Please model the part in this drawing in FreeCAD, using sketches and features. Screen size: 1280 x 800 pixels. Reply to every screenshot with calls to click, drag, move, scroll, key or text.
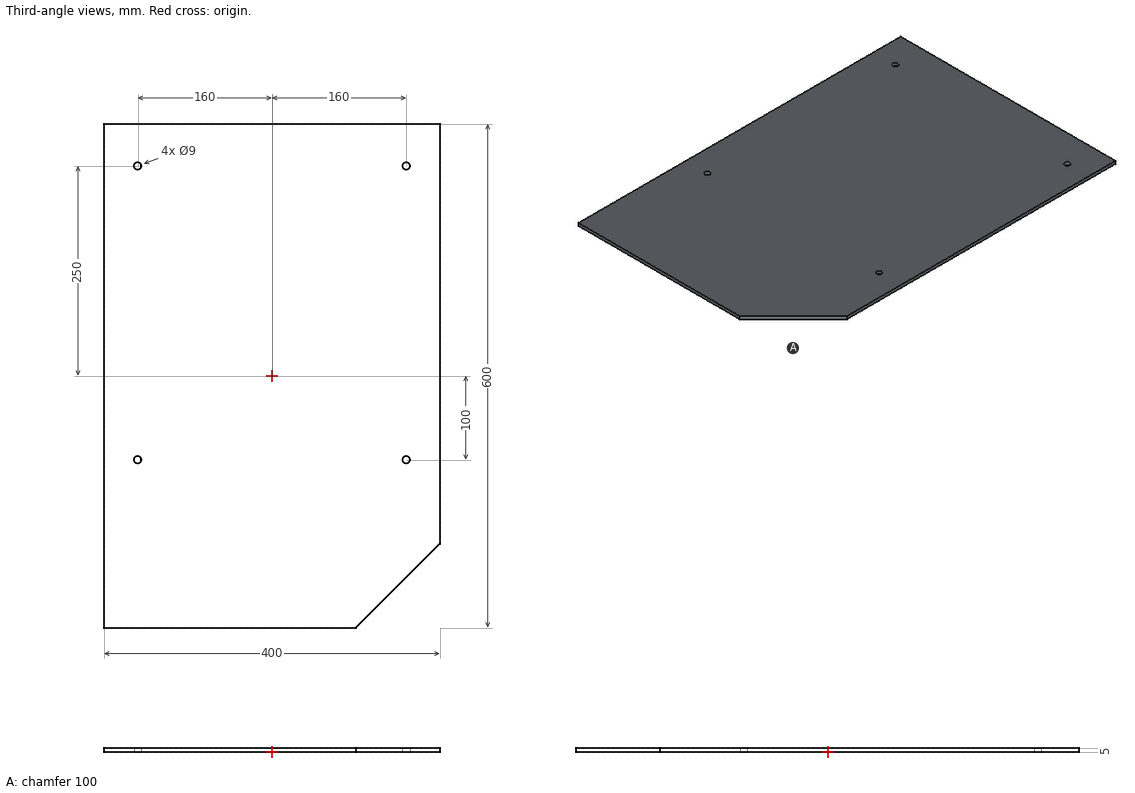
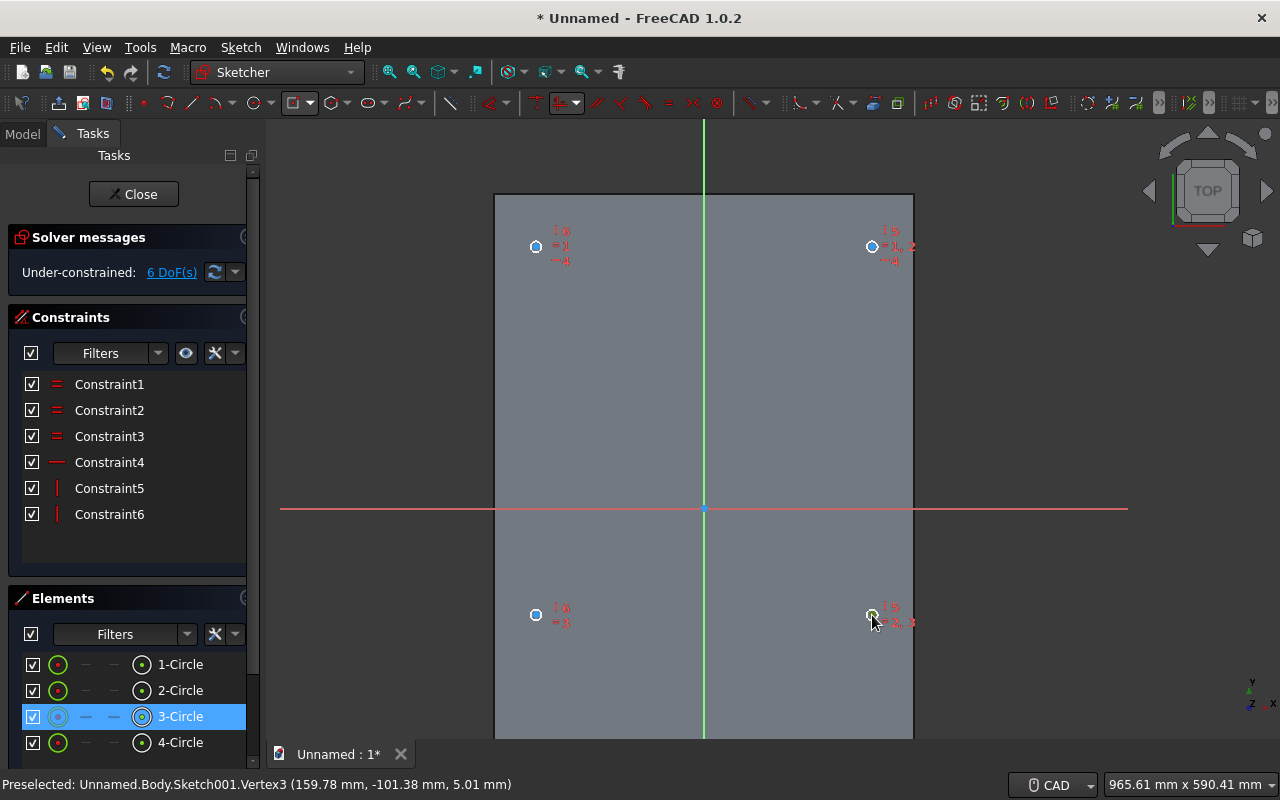
click(536, 615)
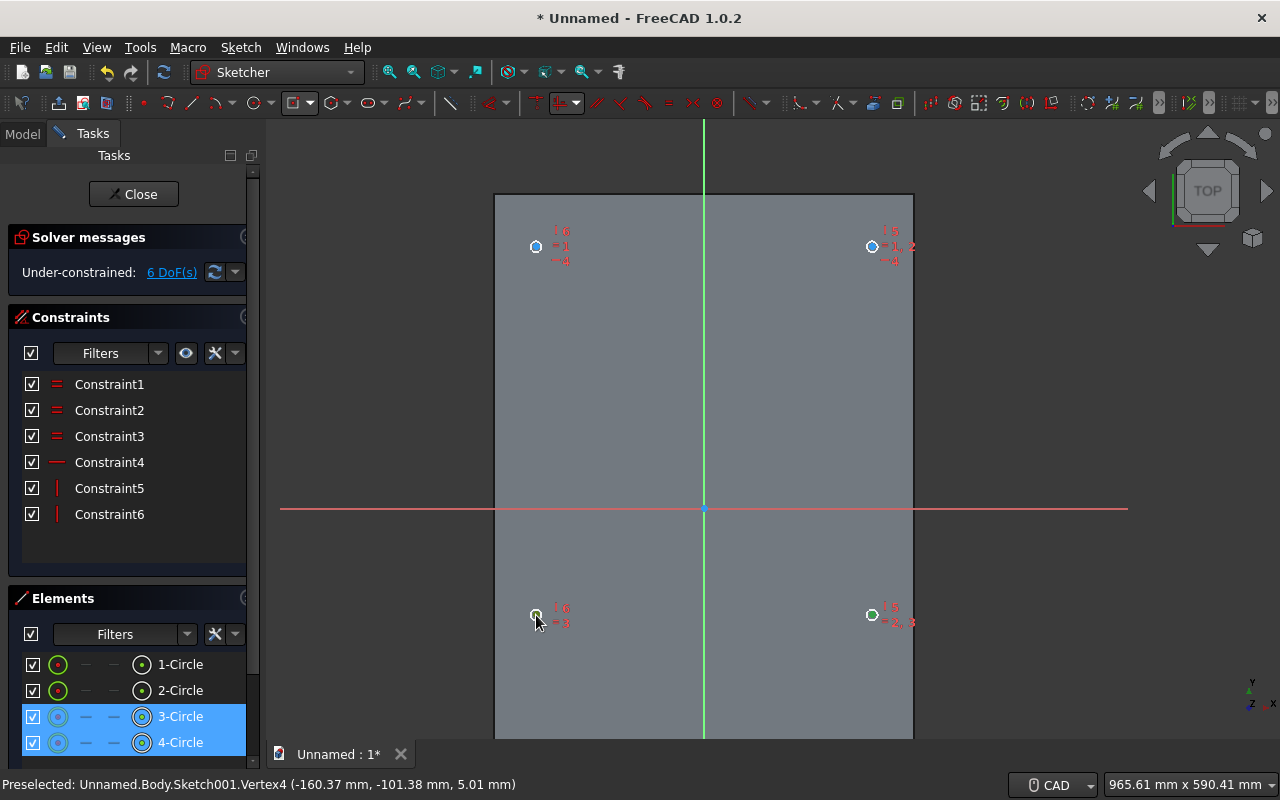
click(578, 104)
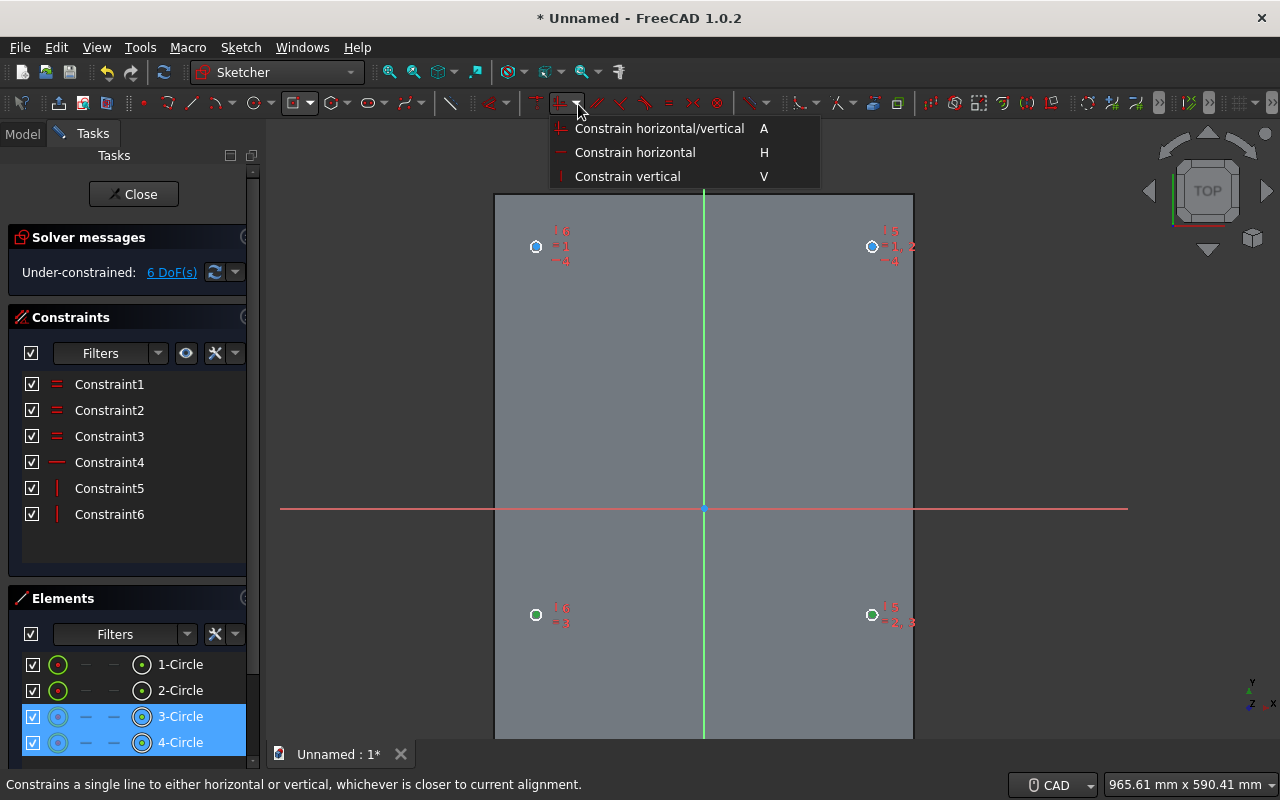
click(685, 152)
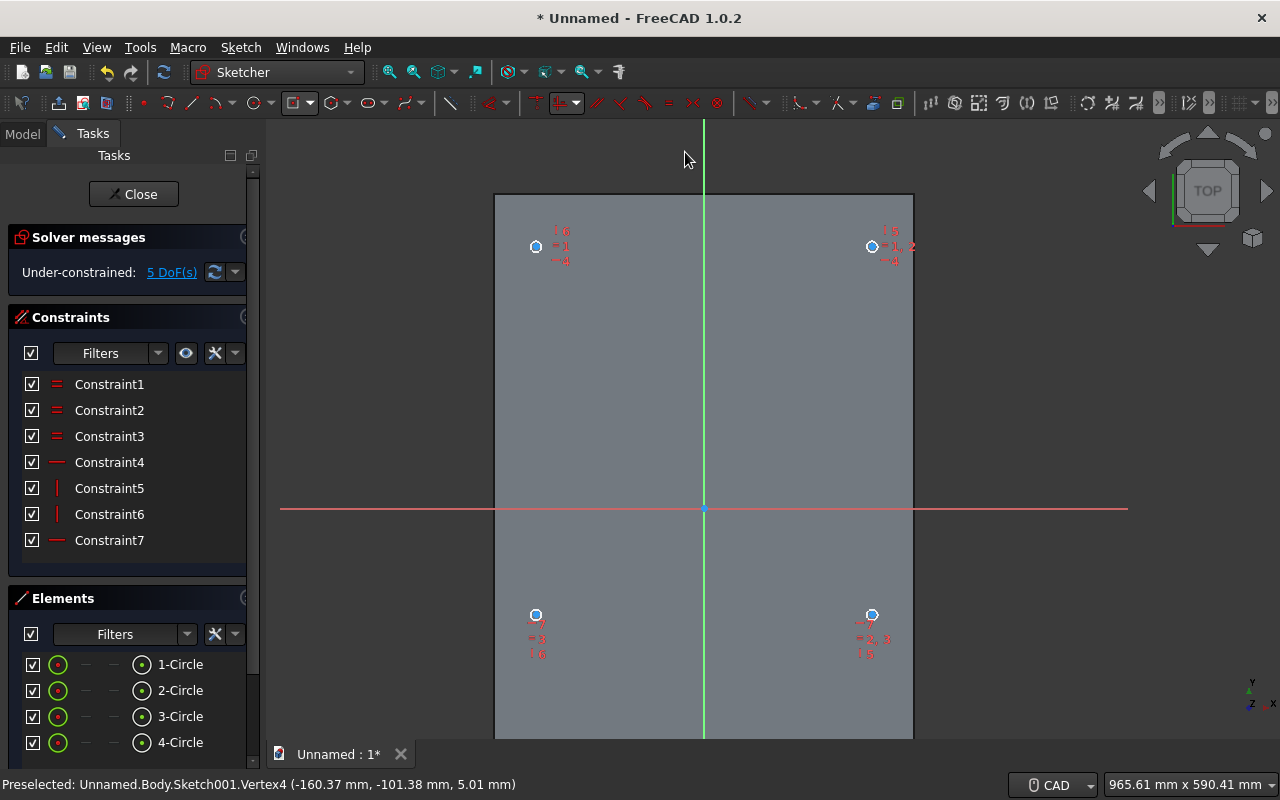
click(490, 104)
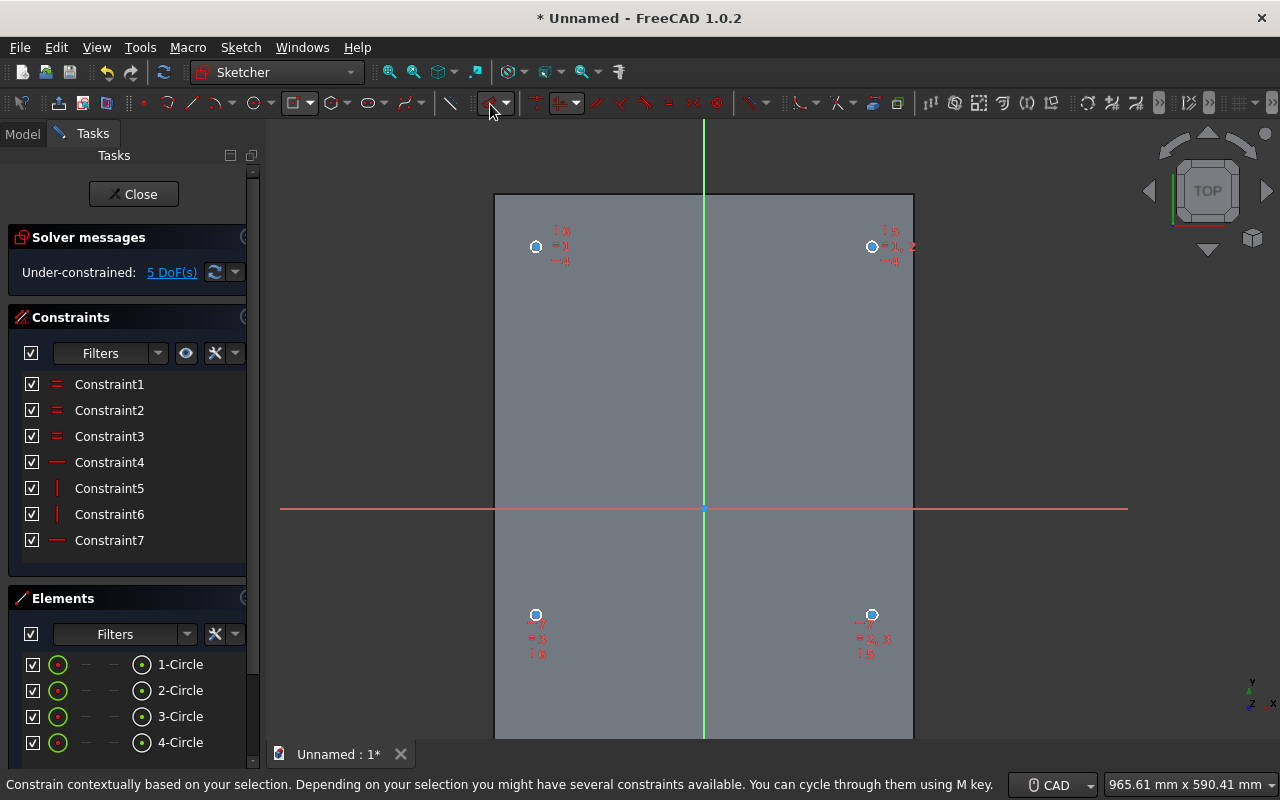
scroll(536, 241, up, 8)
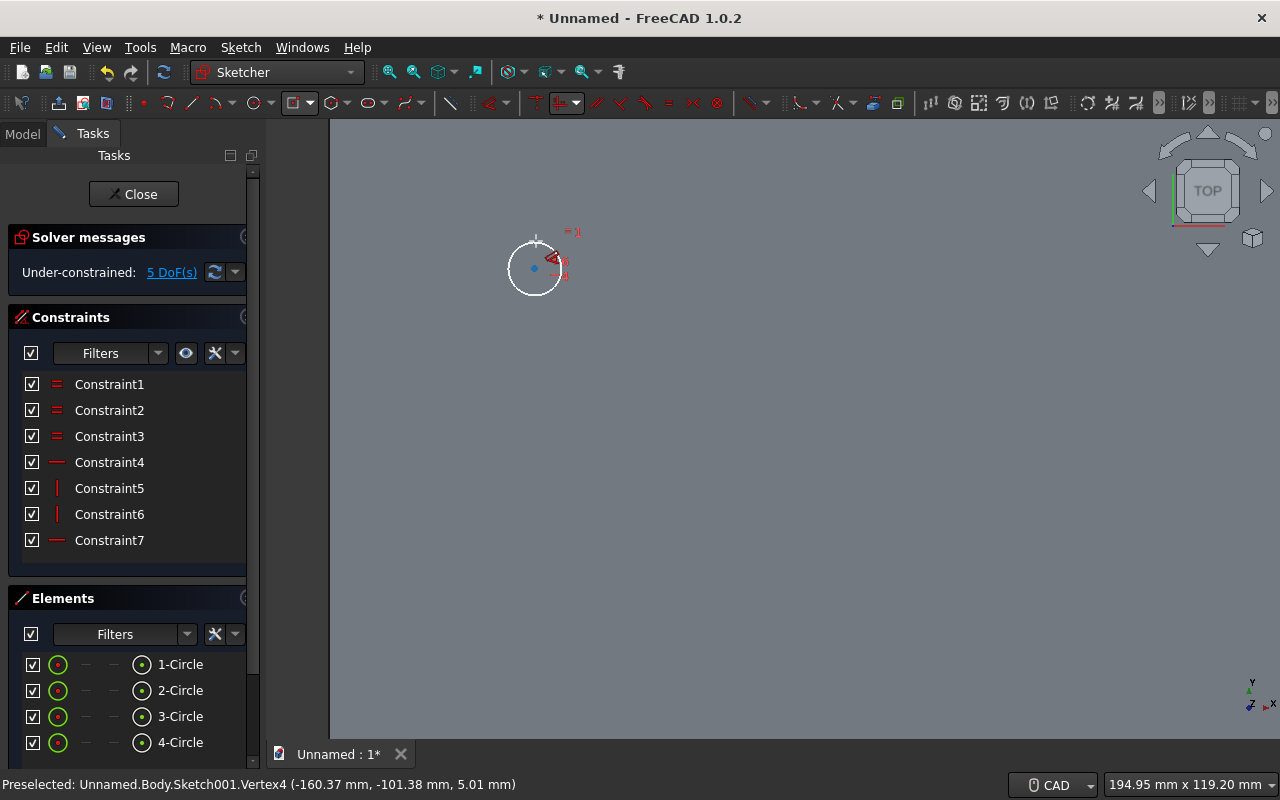
click(536, 242)
click(537, 210)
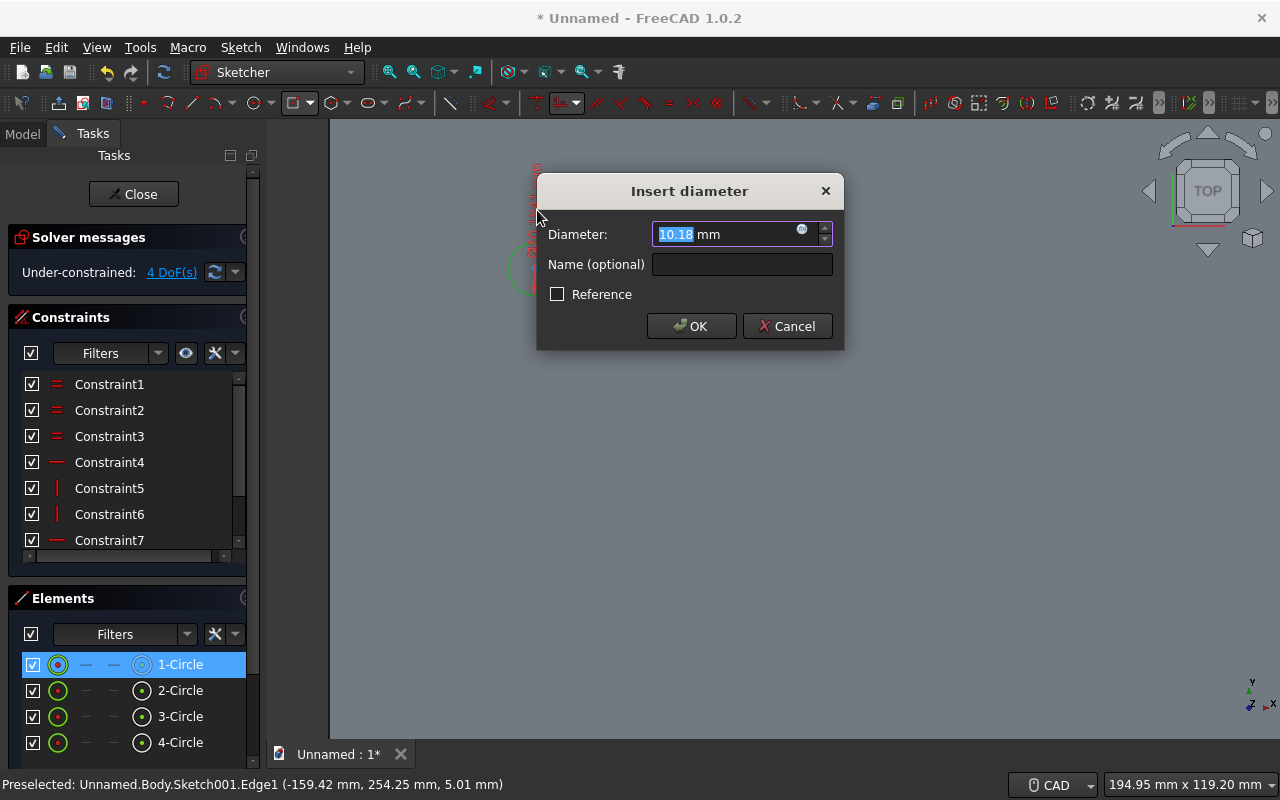
text(9)
key(Return)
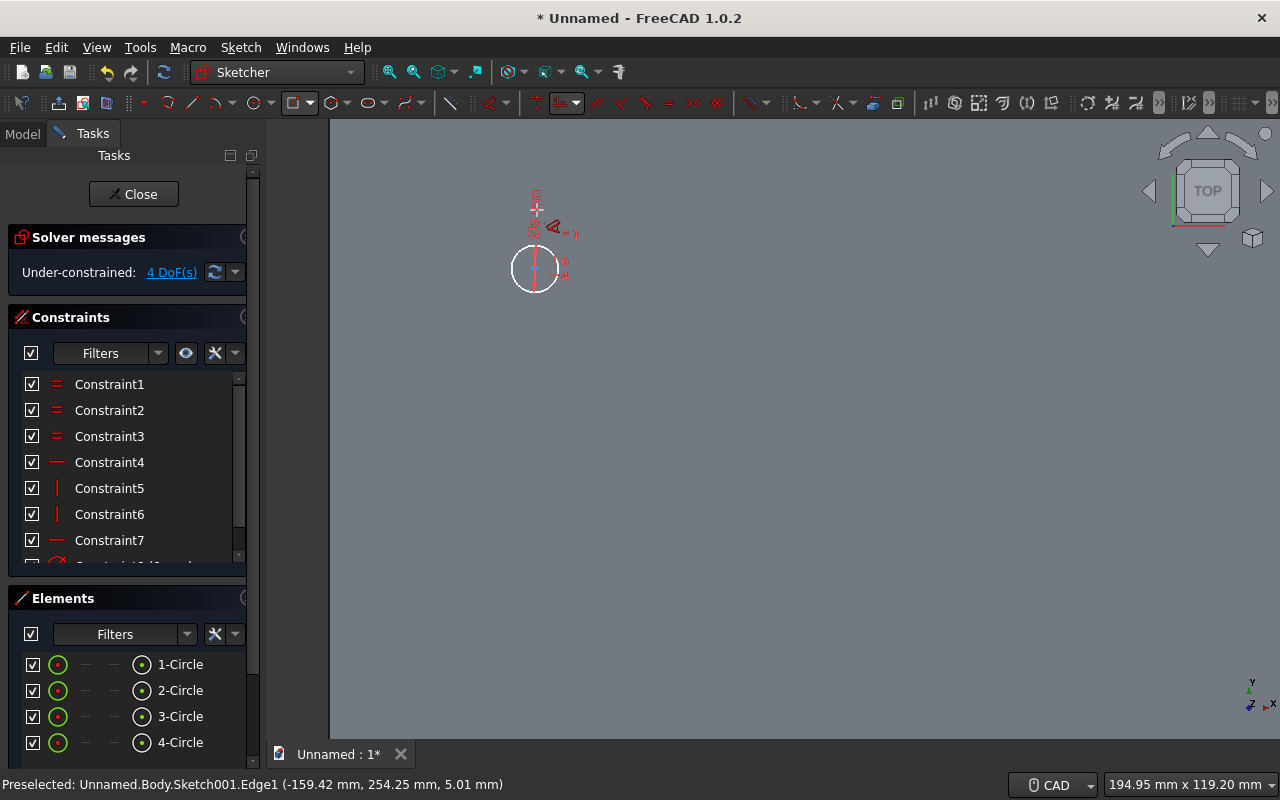
scroll(536, 240, down, 8)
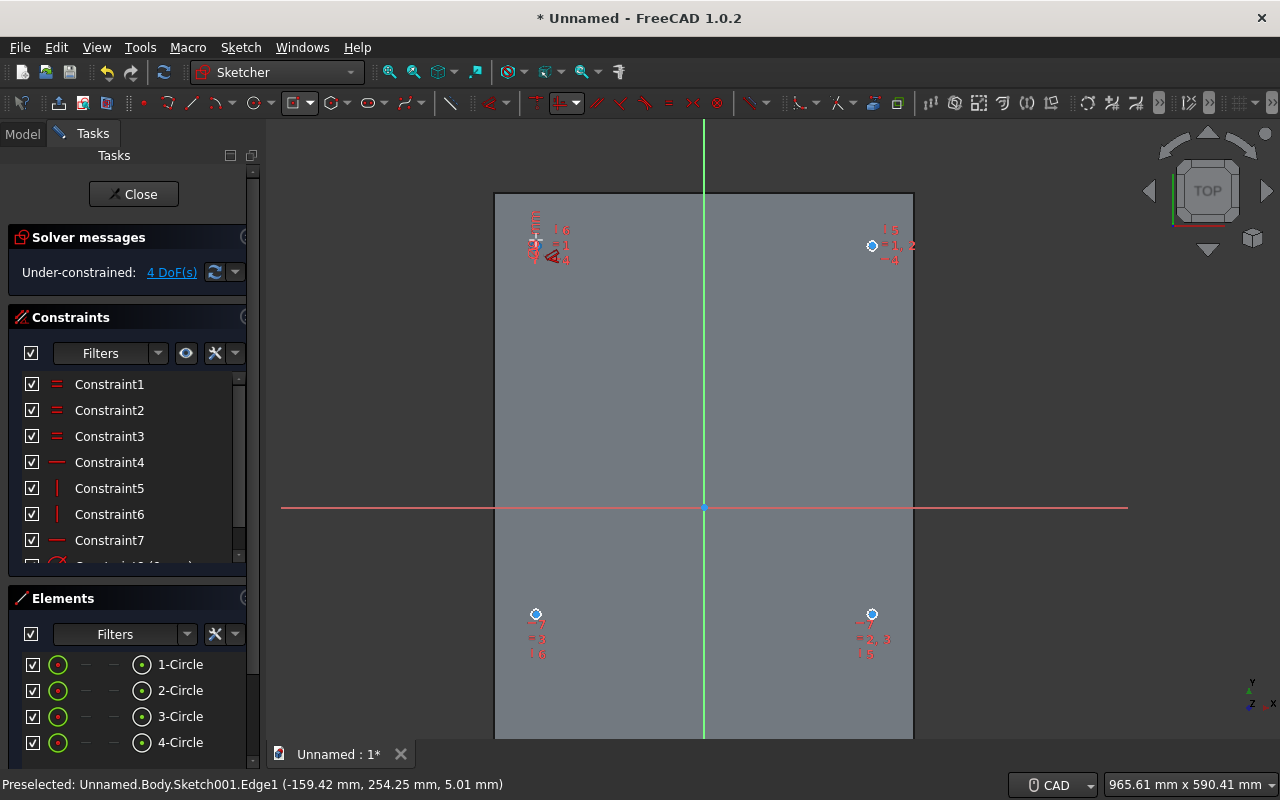
click(536, 246)
click(620, 212)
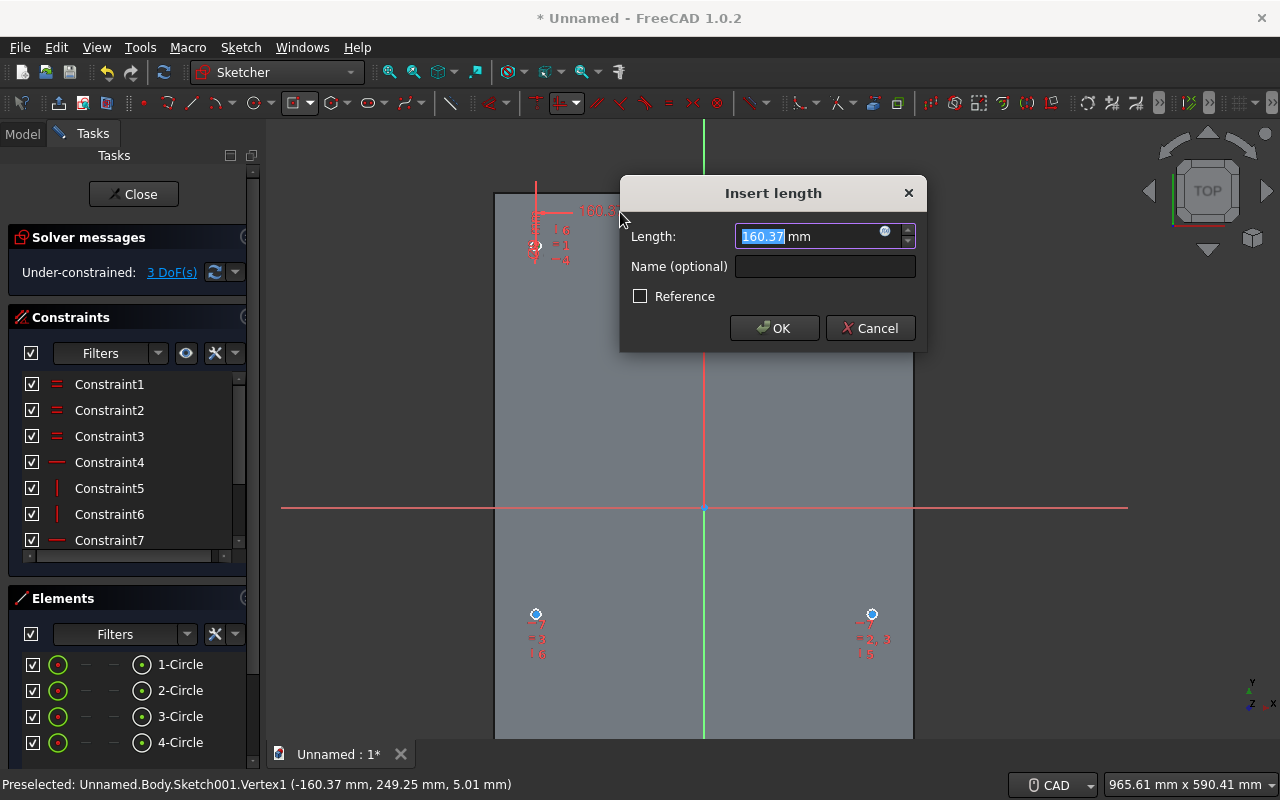
text(160)
key(Return)